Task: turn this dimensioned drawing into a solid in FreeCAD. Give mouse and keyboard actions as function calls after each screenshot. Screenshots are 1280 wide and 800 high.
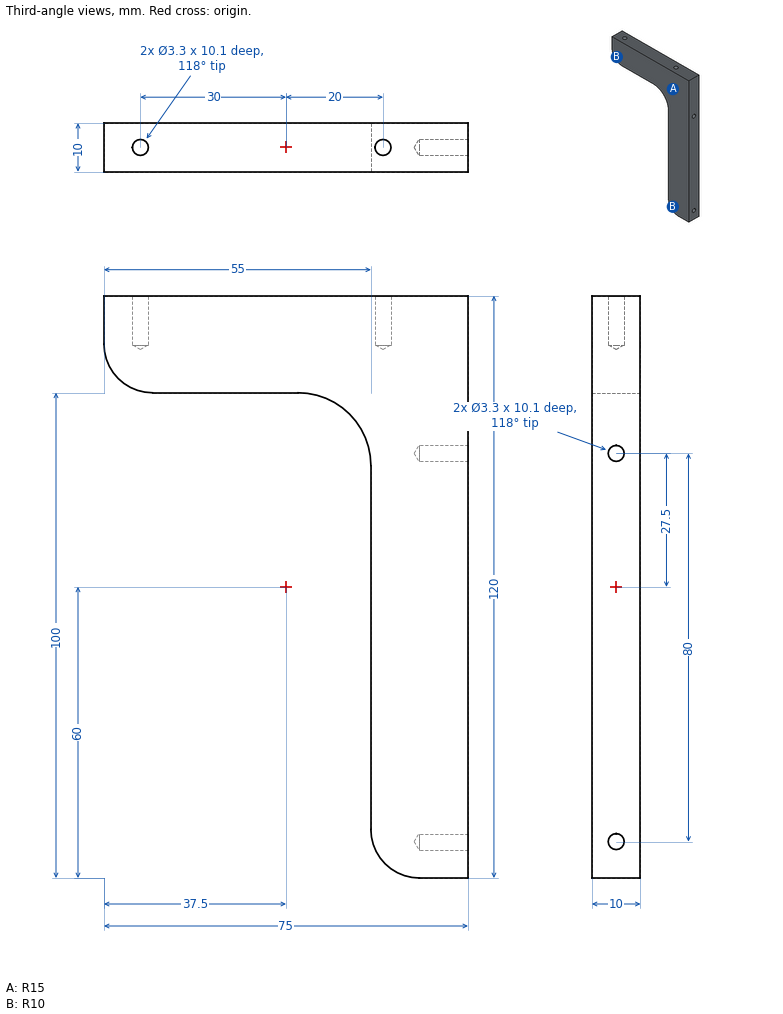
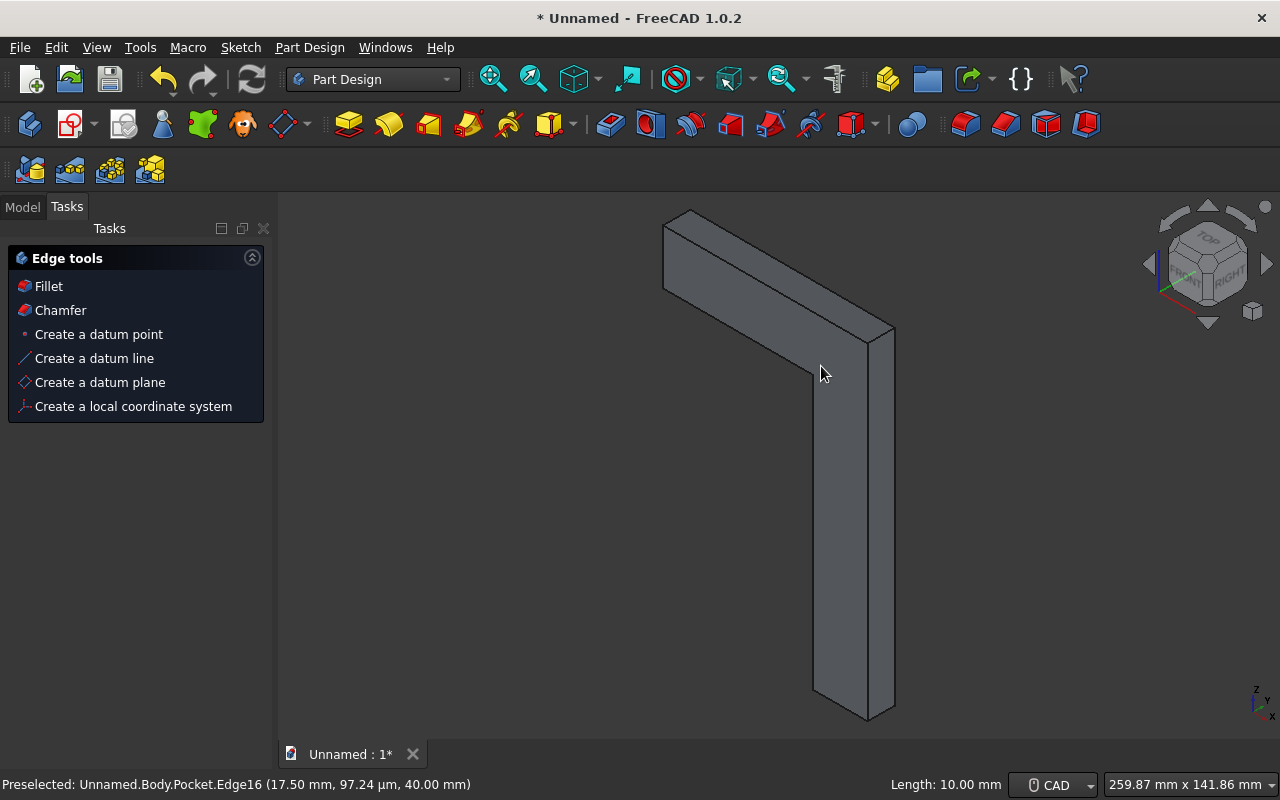
click(966, 124)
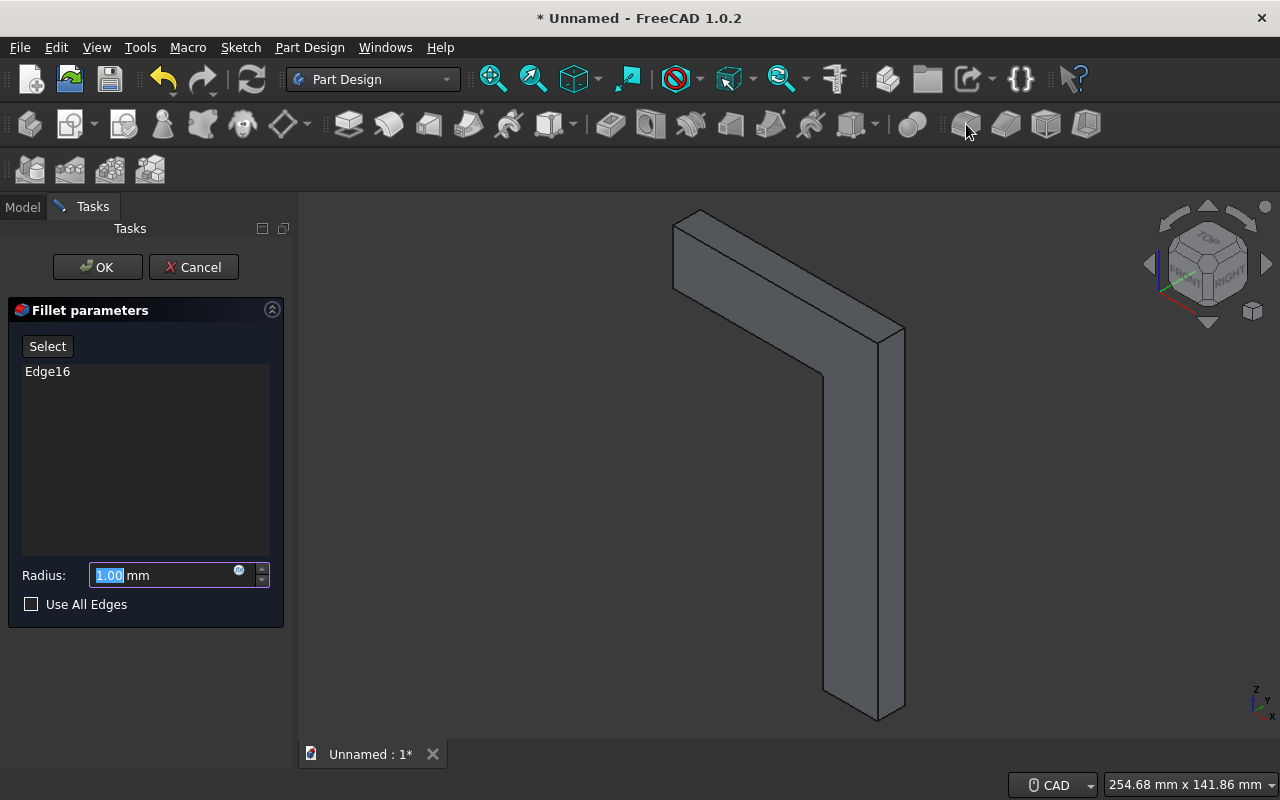
text(15)
key(Tab)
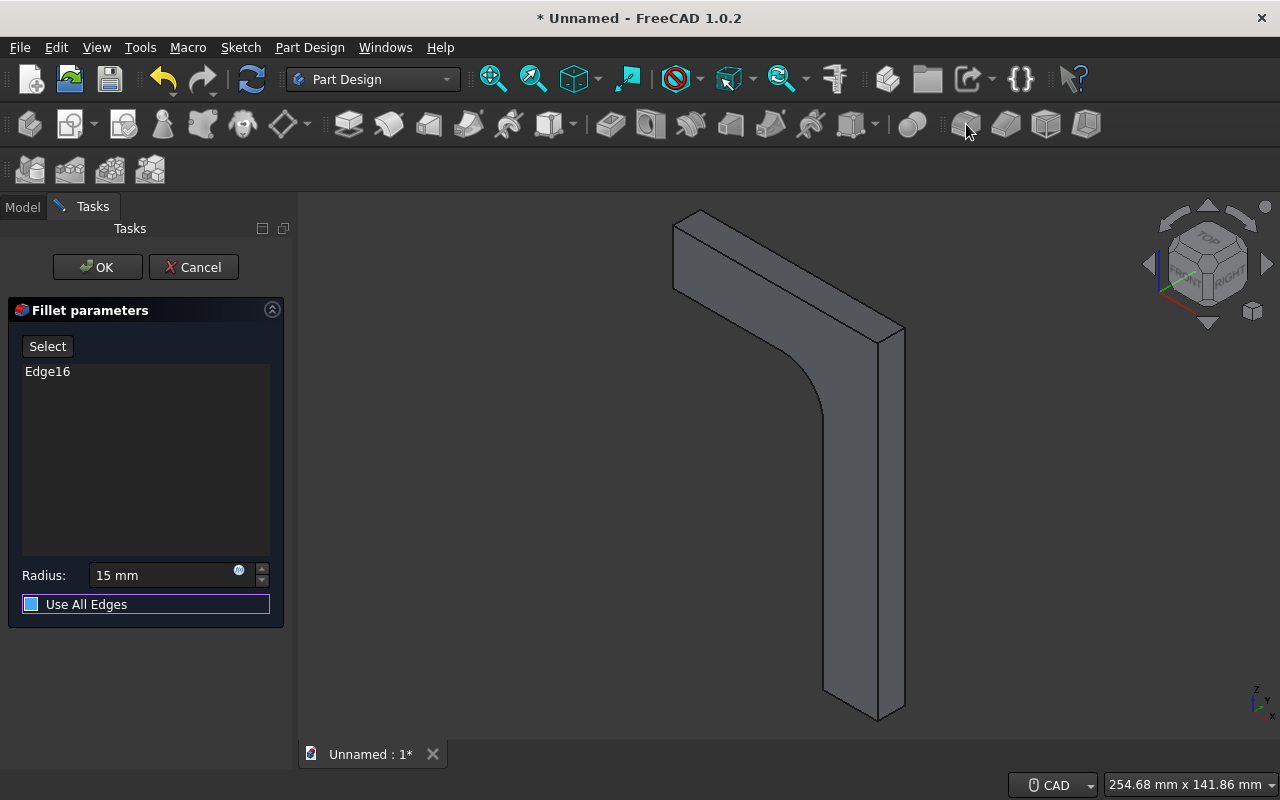
click(98, 267)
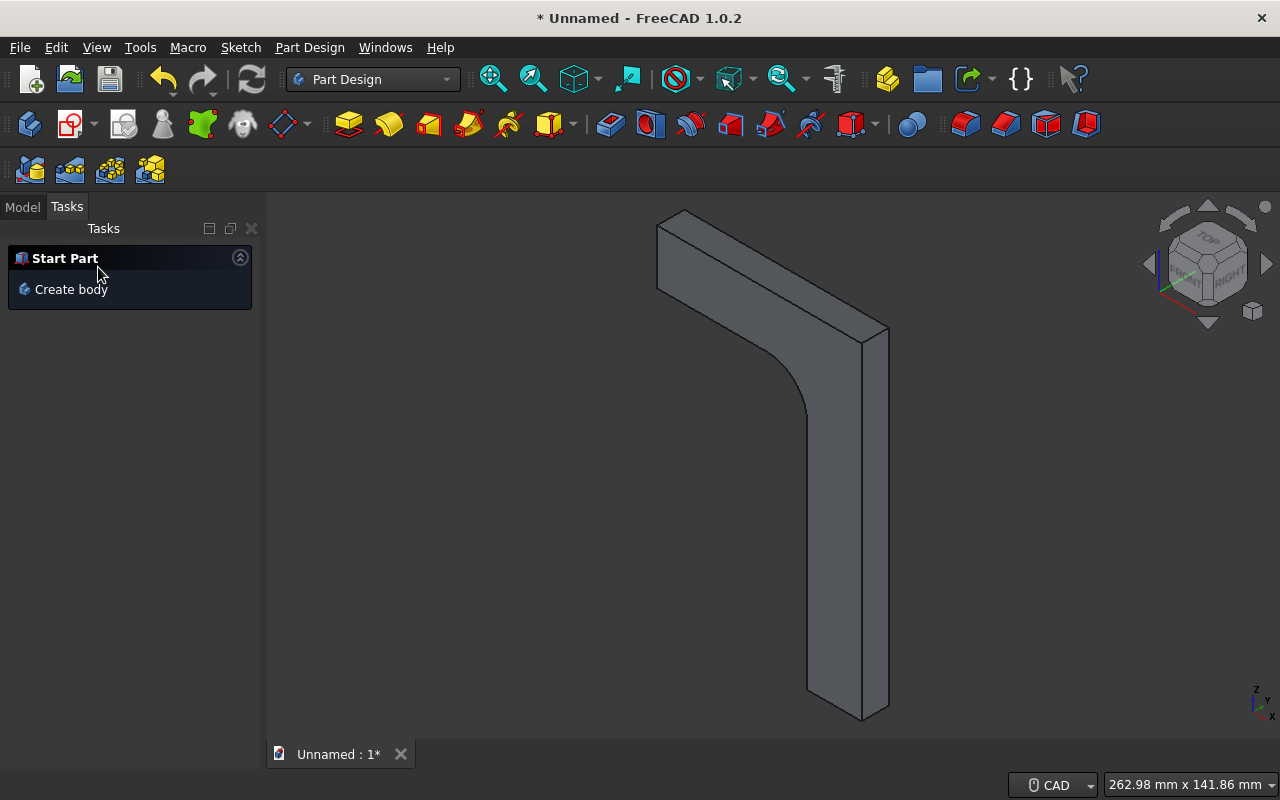
key(2)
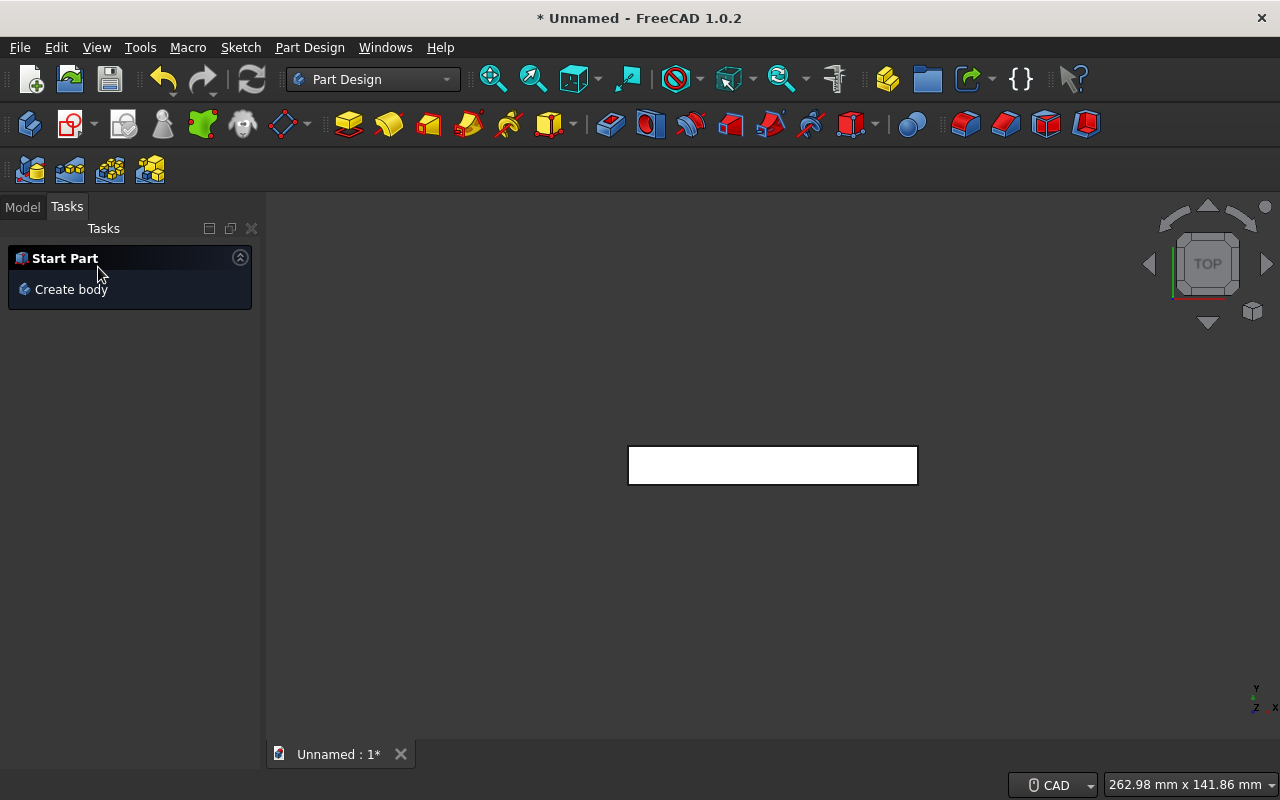
key(v)
key(f)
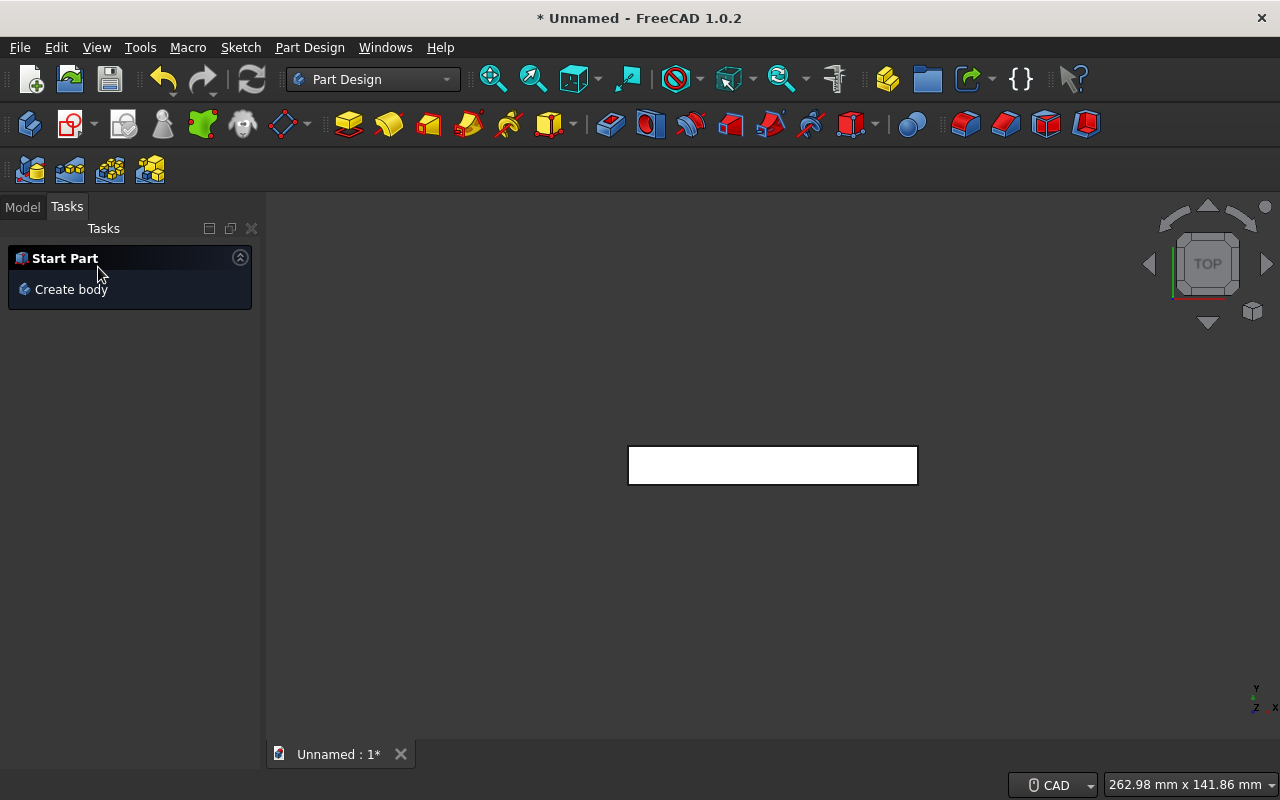
key(0)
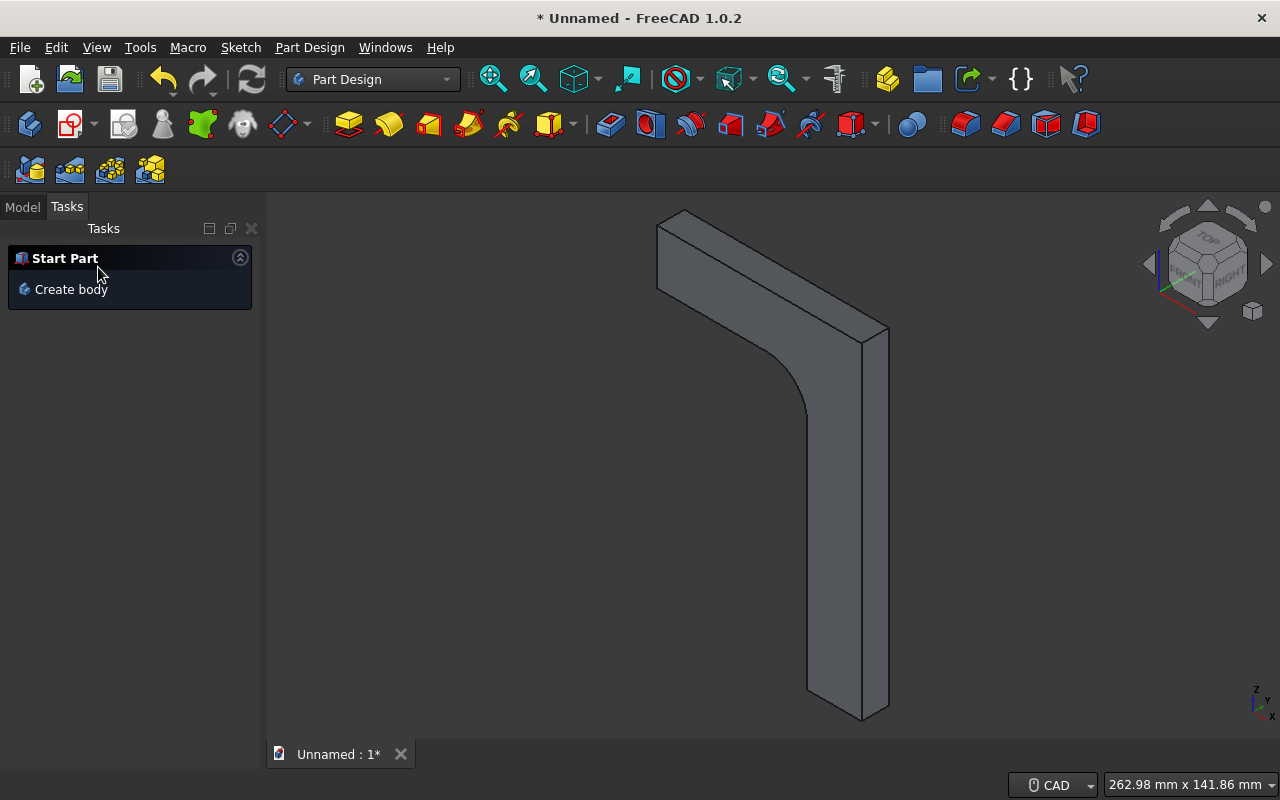
key(1)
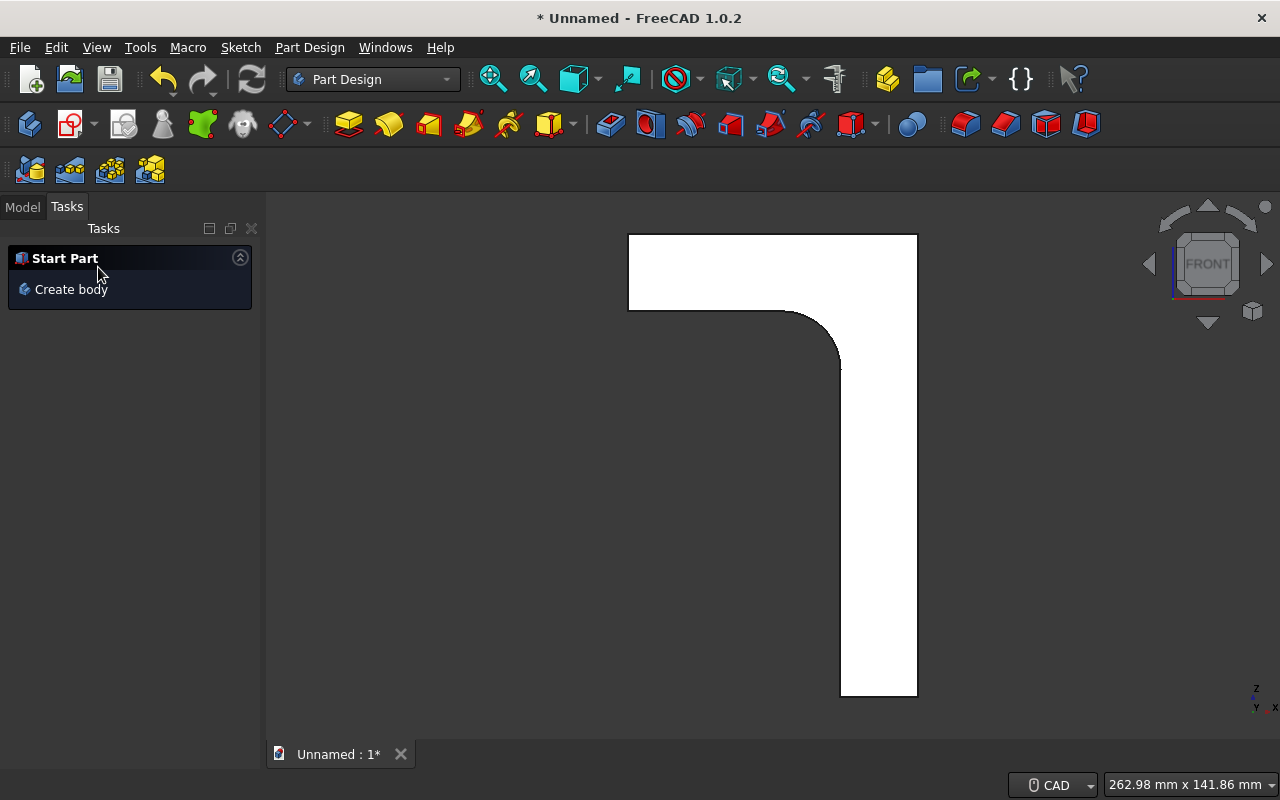
key(3)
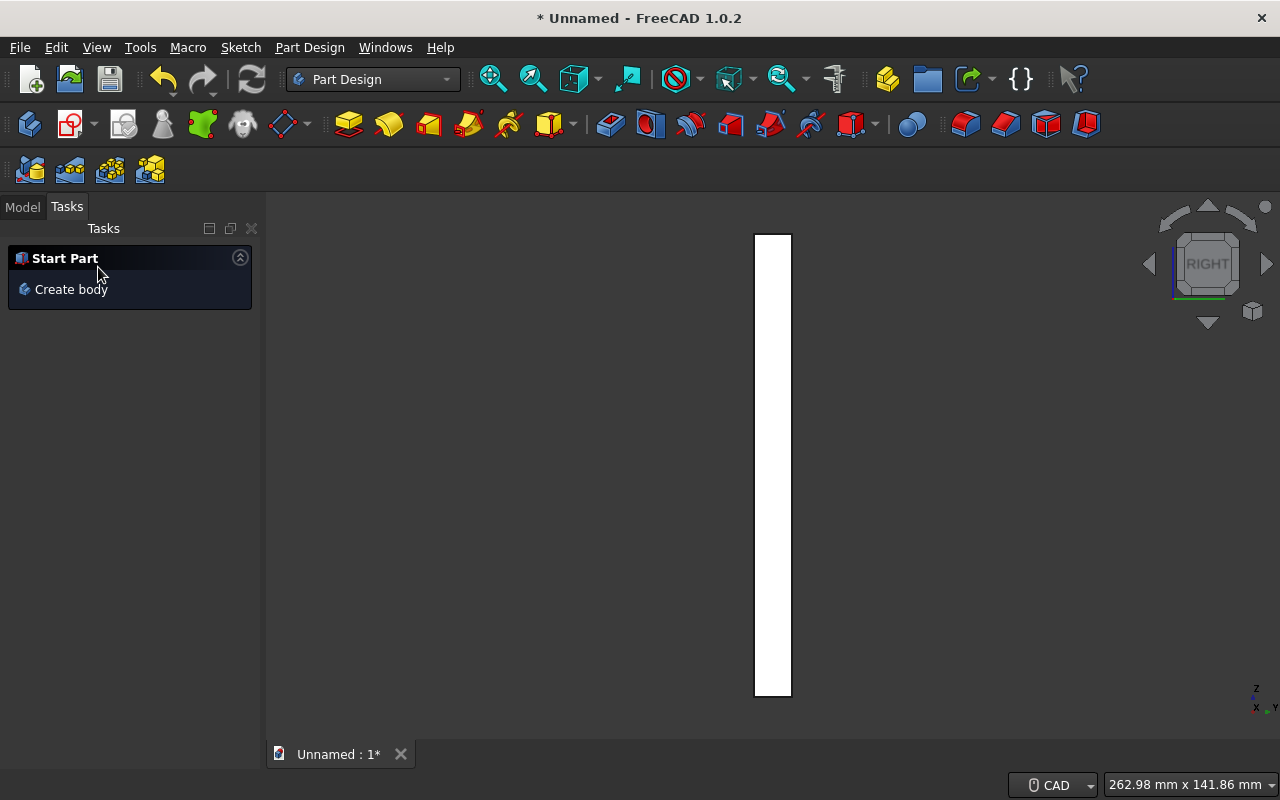
key(5)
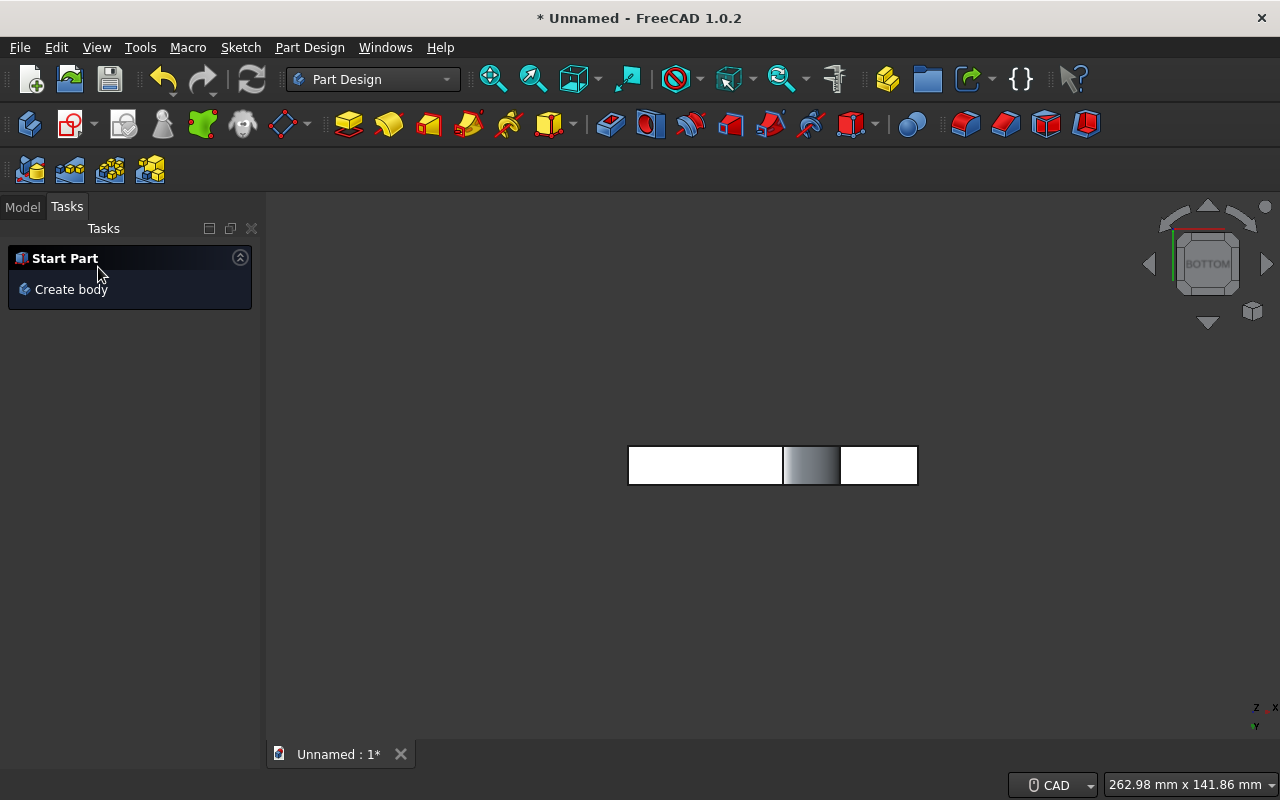
key(v)
key(f)